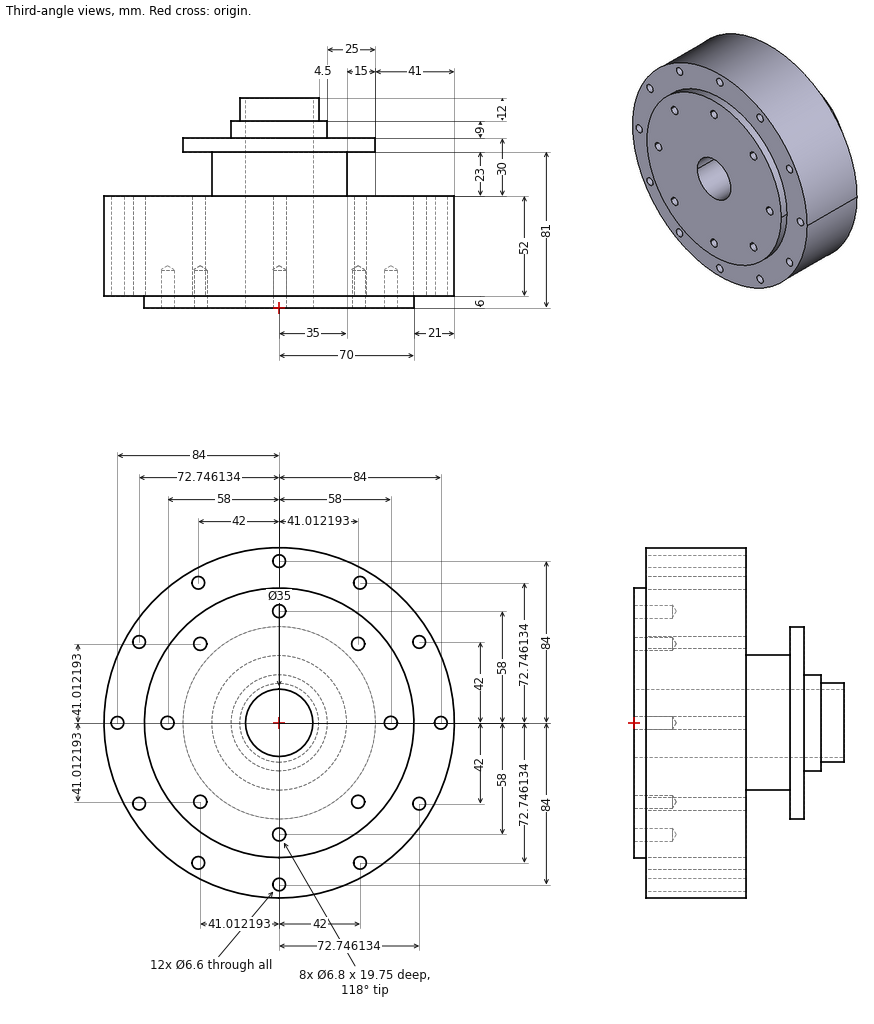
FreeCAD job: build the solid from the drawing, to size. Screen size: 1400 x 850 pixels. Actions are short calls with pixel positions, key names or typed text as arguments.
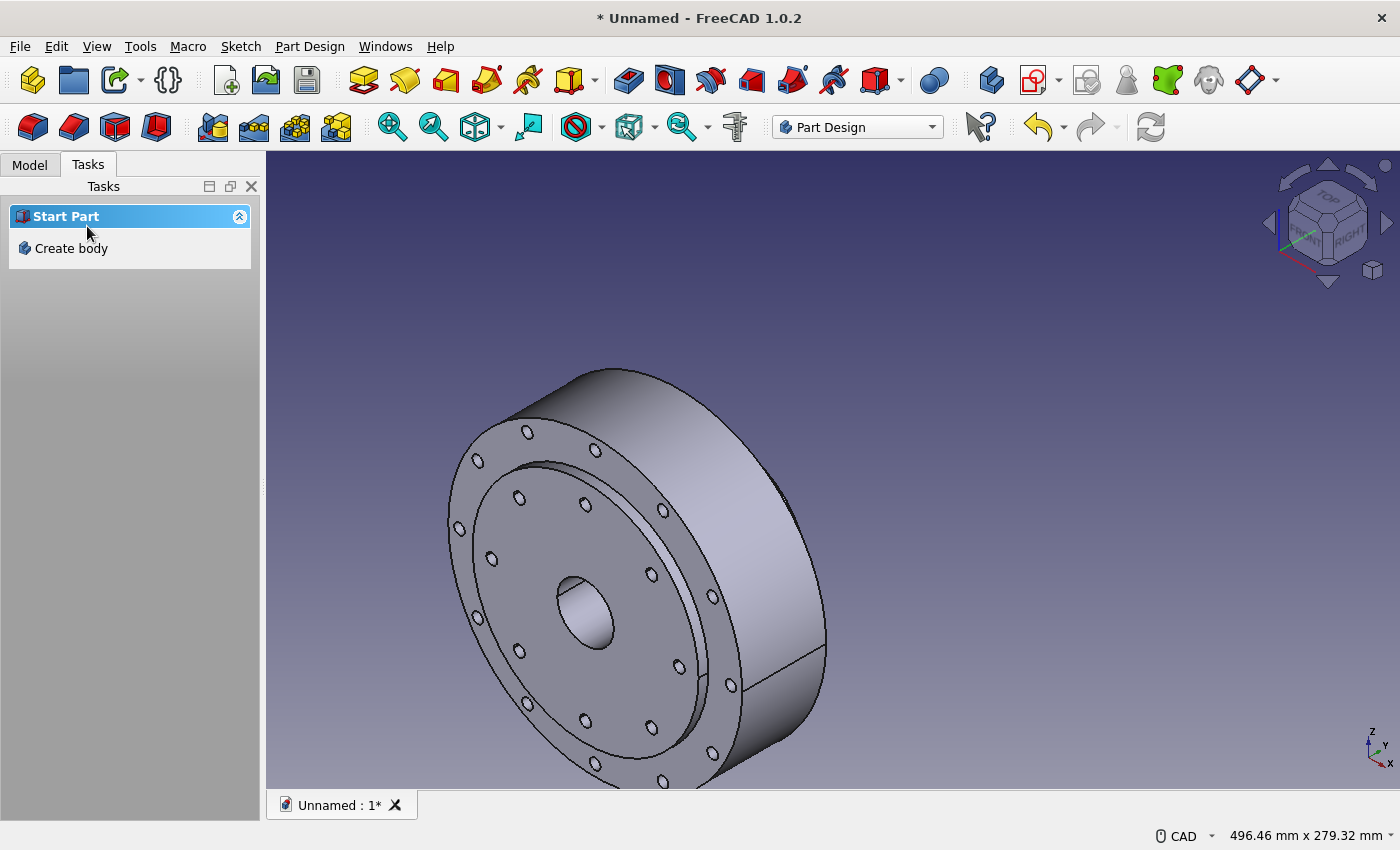
key(v)
key(f)